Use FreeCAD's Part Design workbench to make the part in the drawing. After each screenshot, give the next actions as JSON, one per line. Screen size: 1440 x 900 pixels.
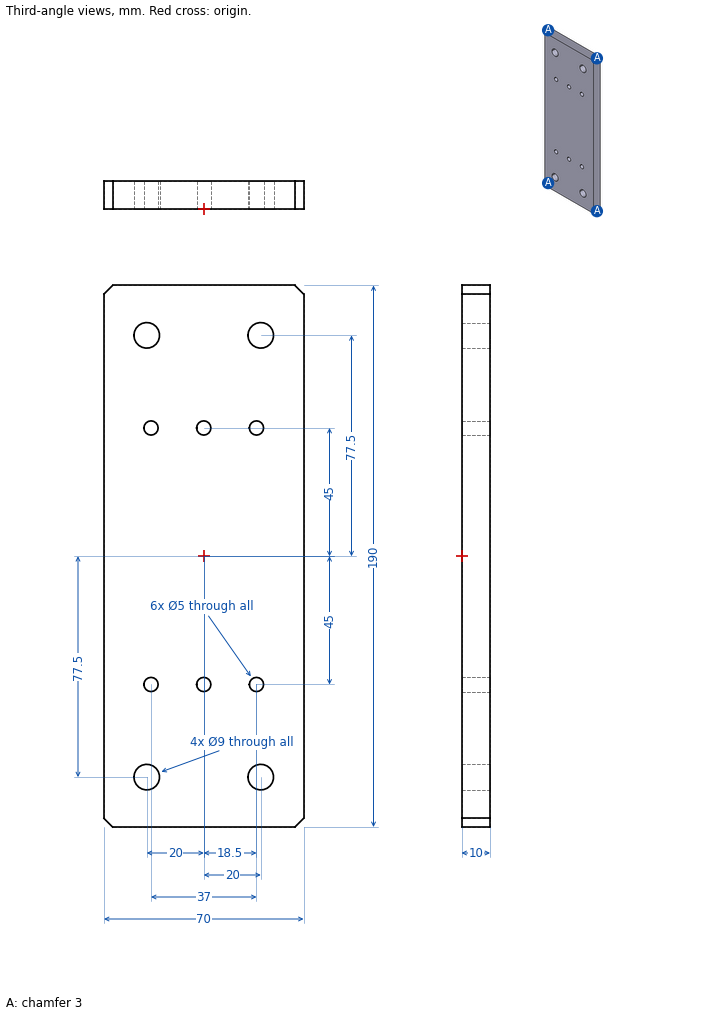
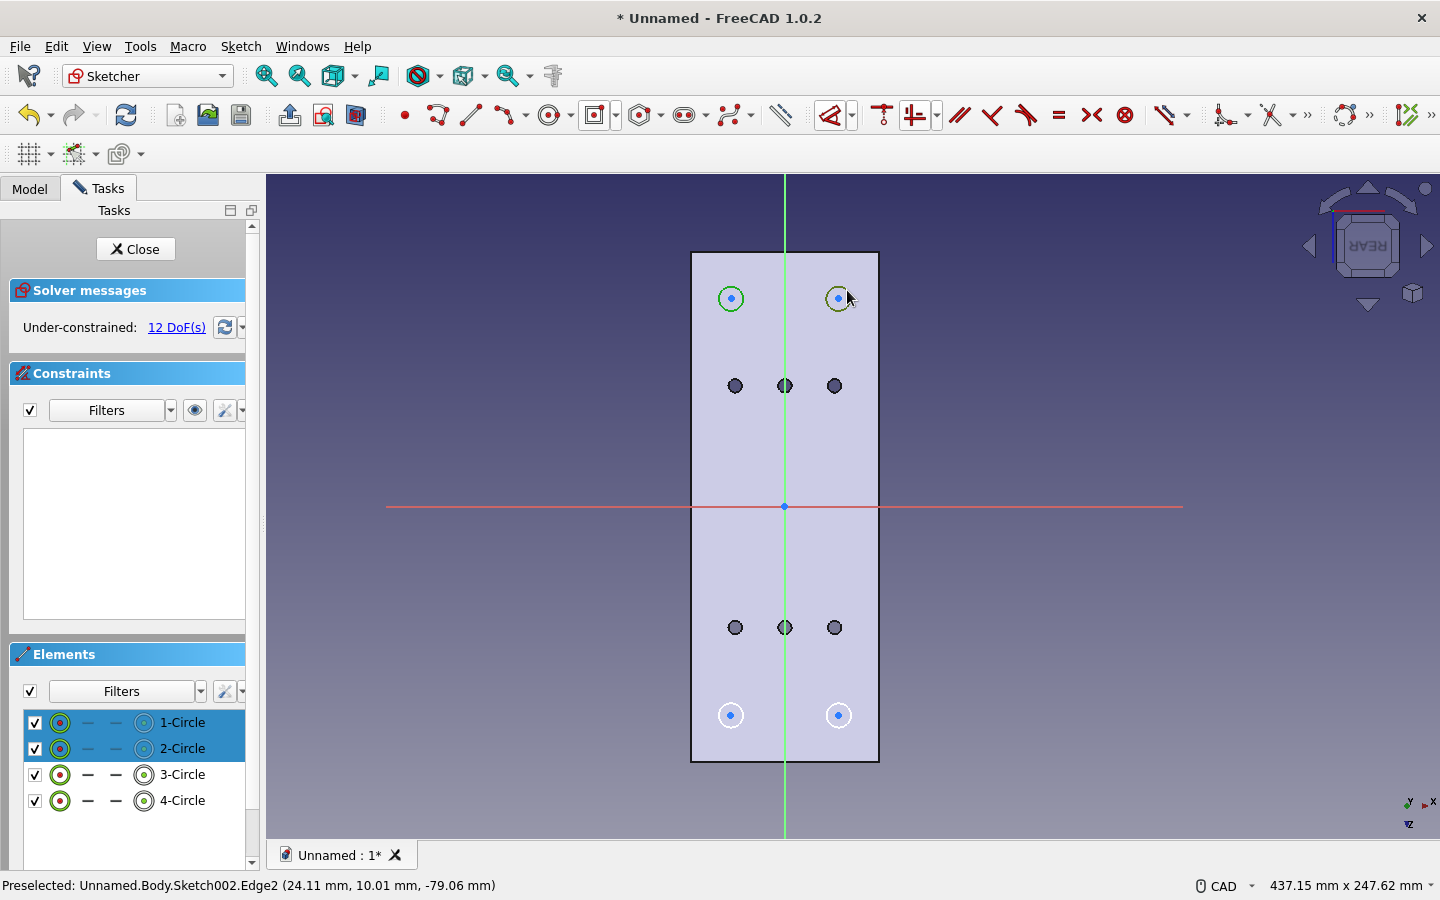
{"action": "left_click", "coordinate": [847, 707]}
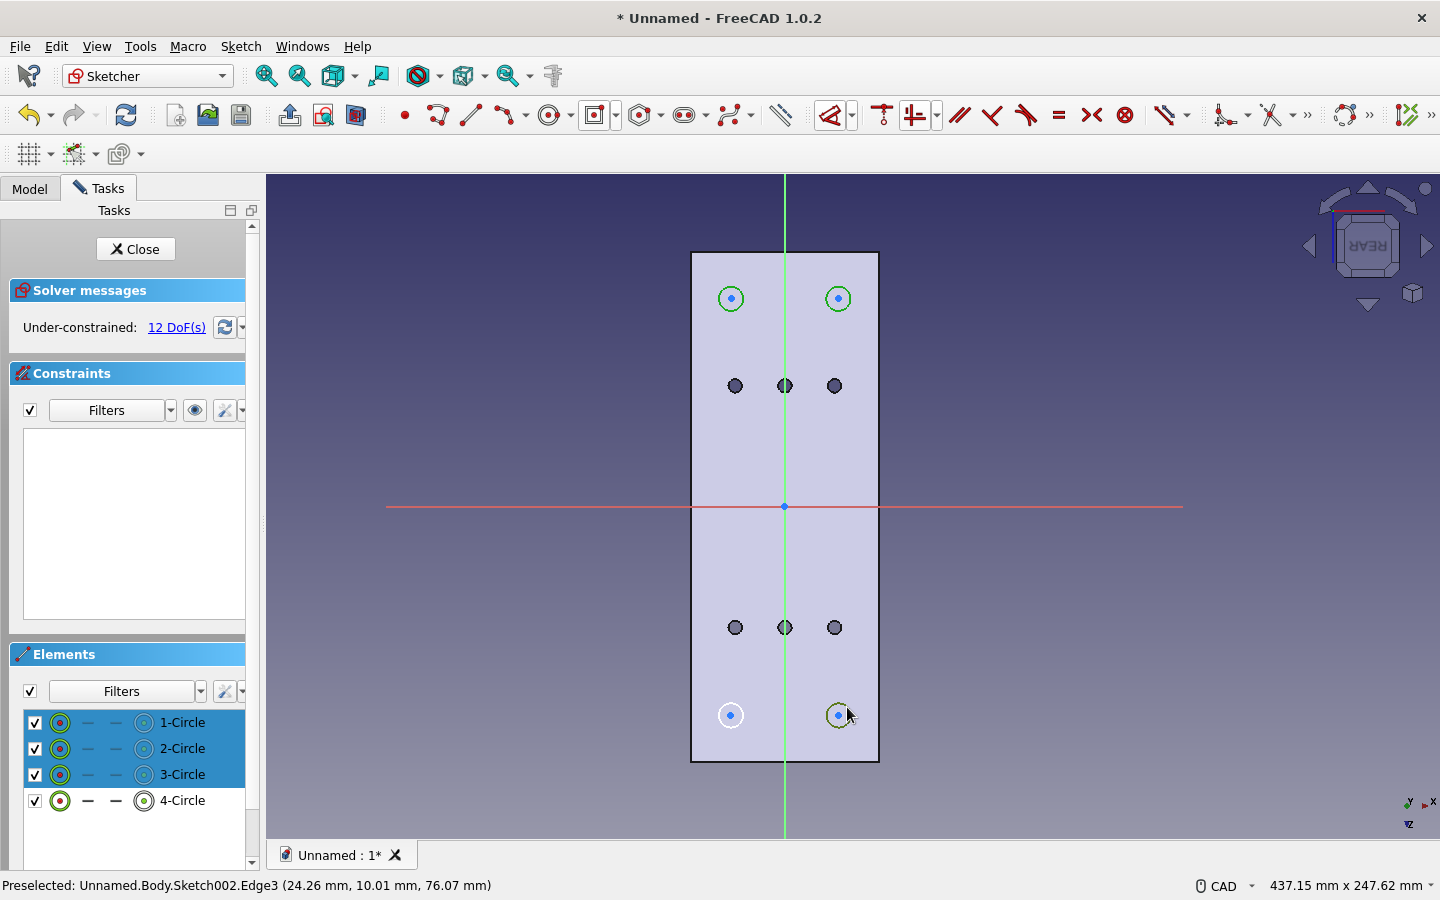
{"action": "left_click", "coordinate": [739, 707]}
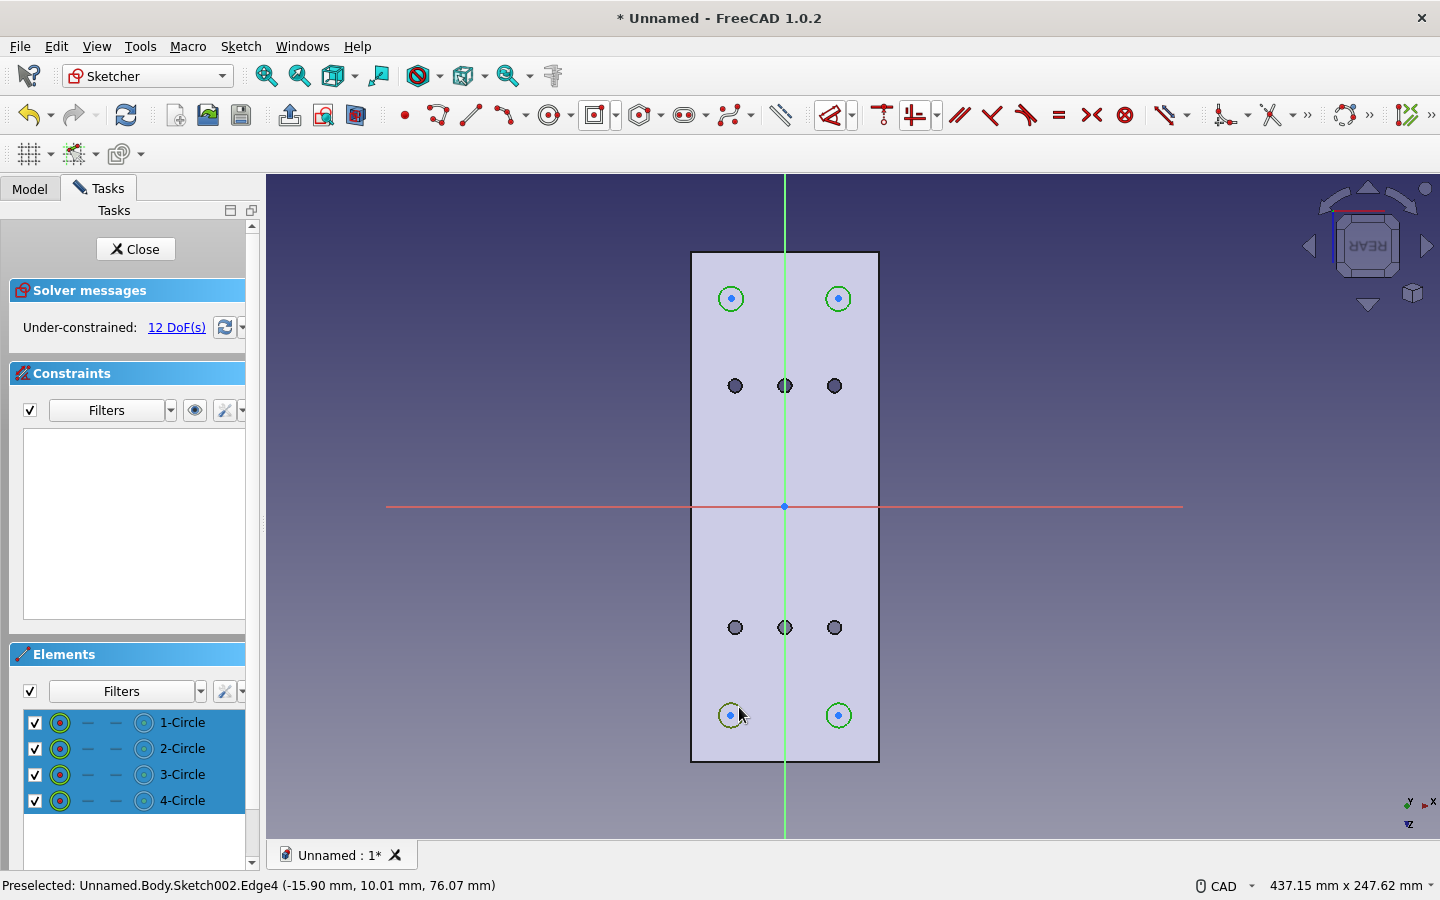
{"action": "left_click", "coordinate": [1059, 116]}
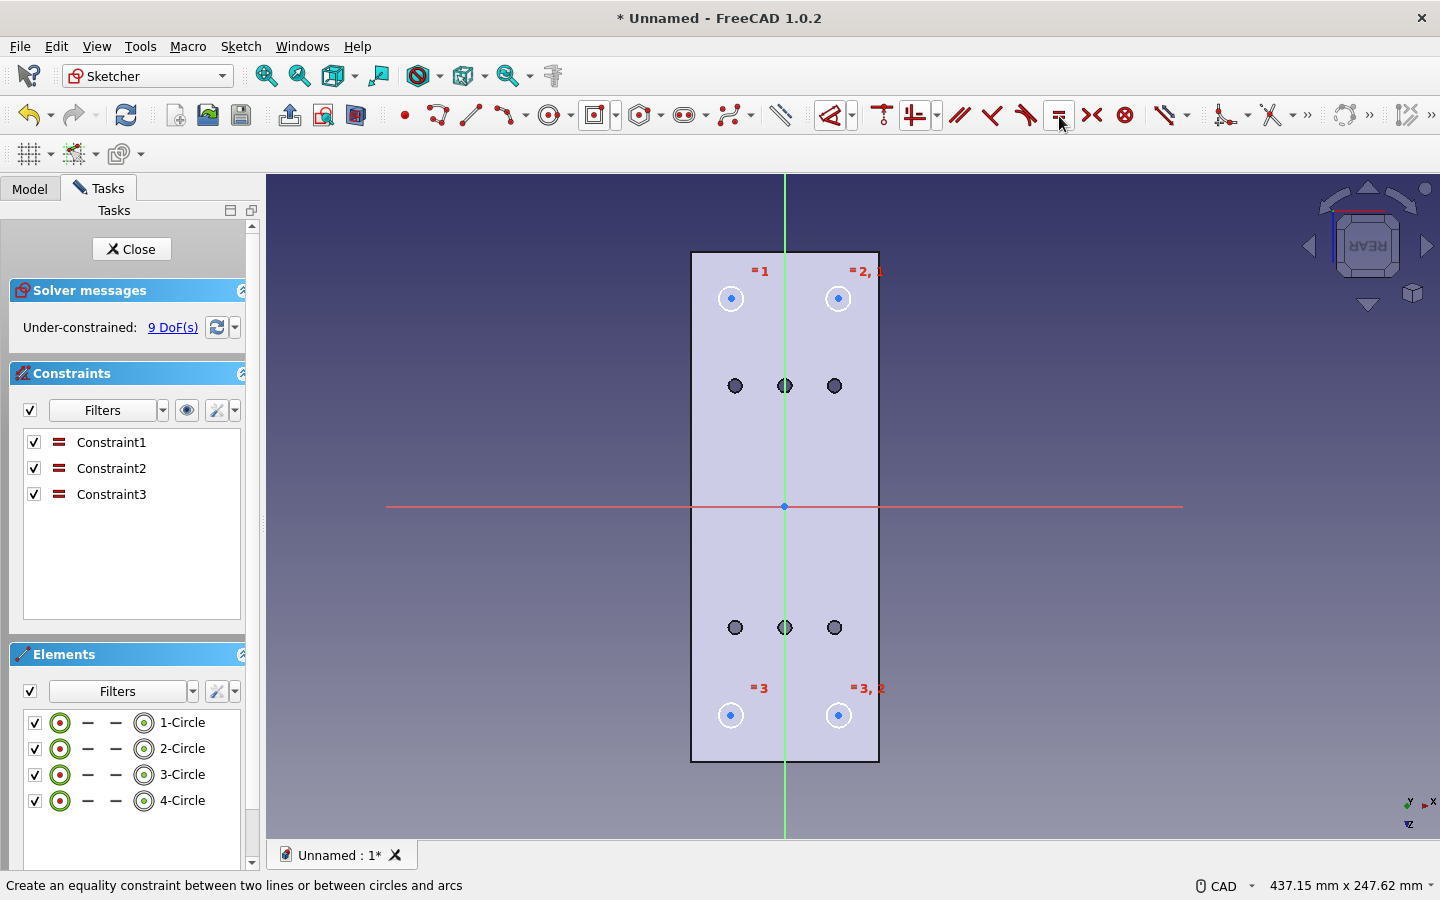
{"action": "left_click", "coordinate": [731, 299]}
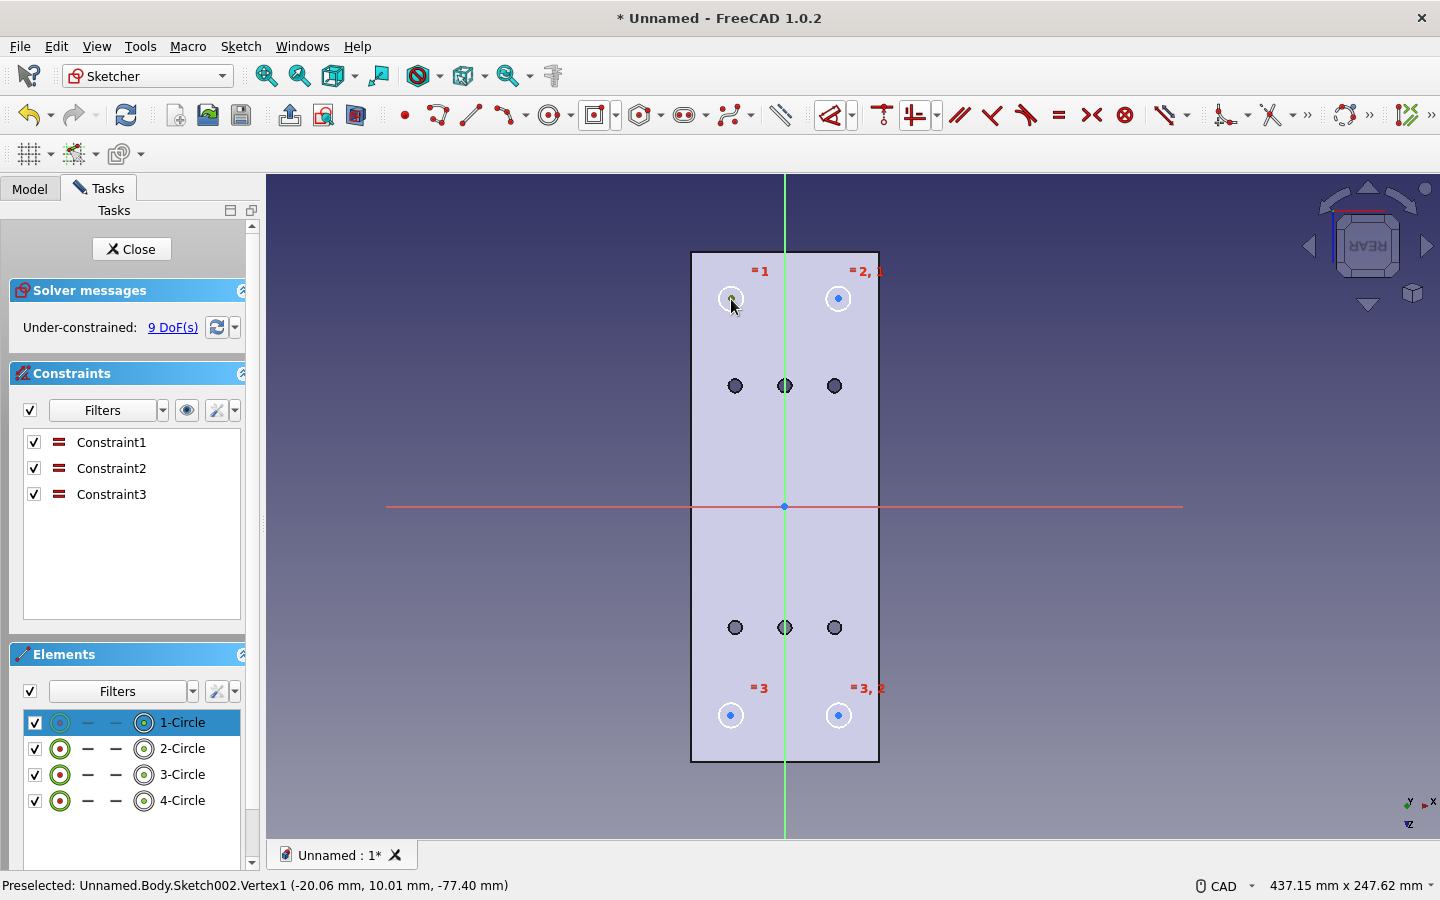
{"action": "left_click", "coordinate": [838, 299]}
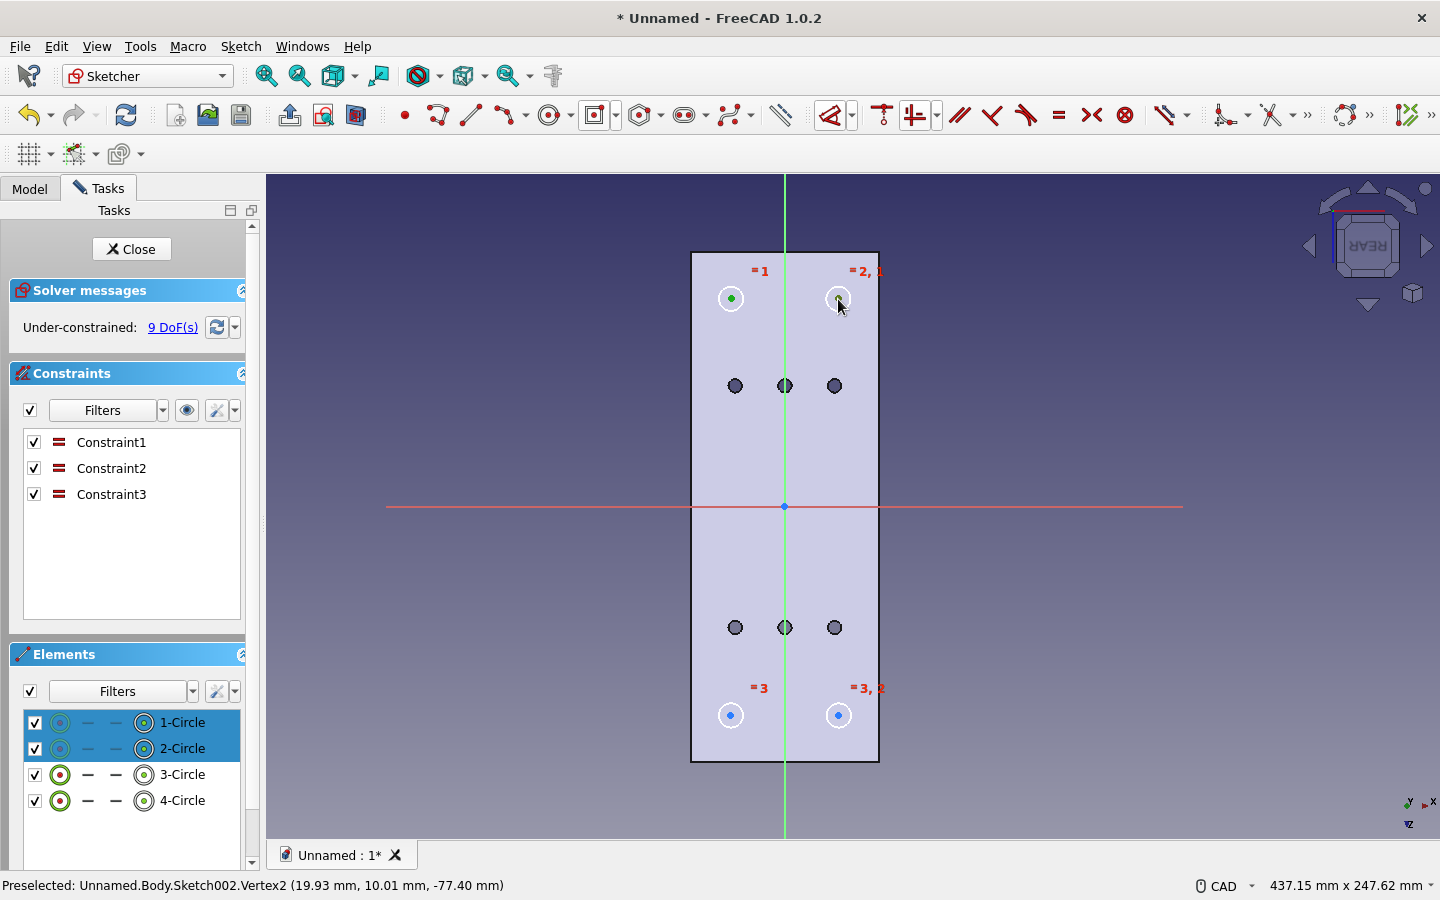
{"action": "key", "text": "h"}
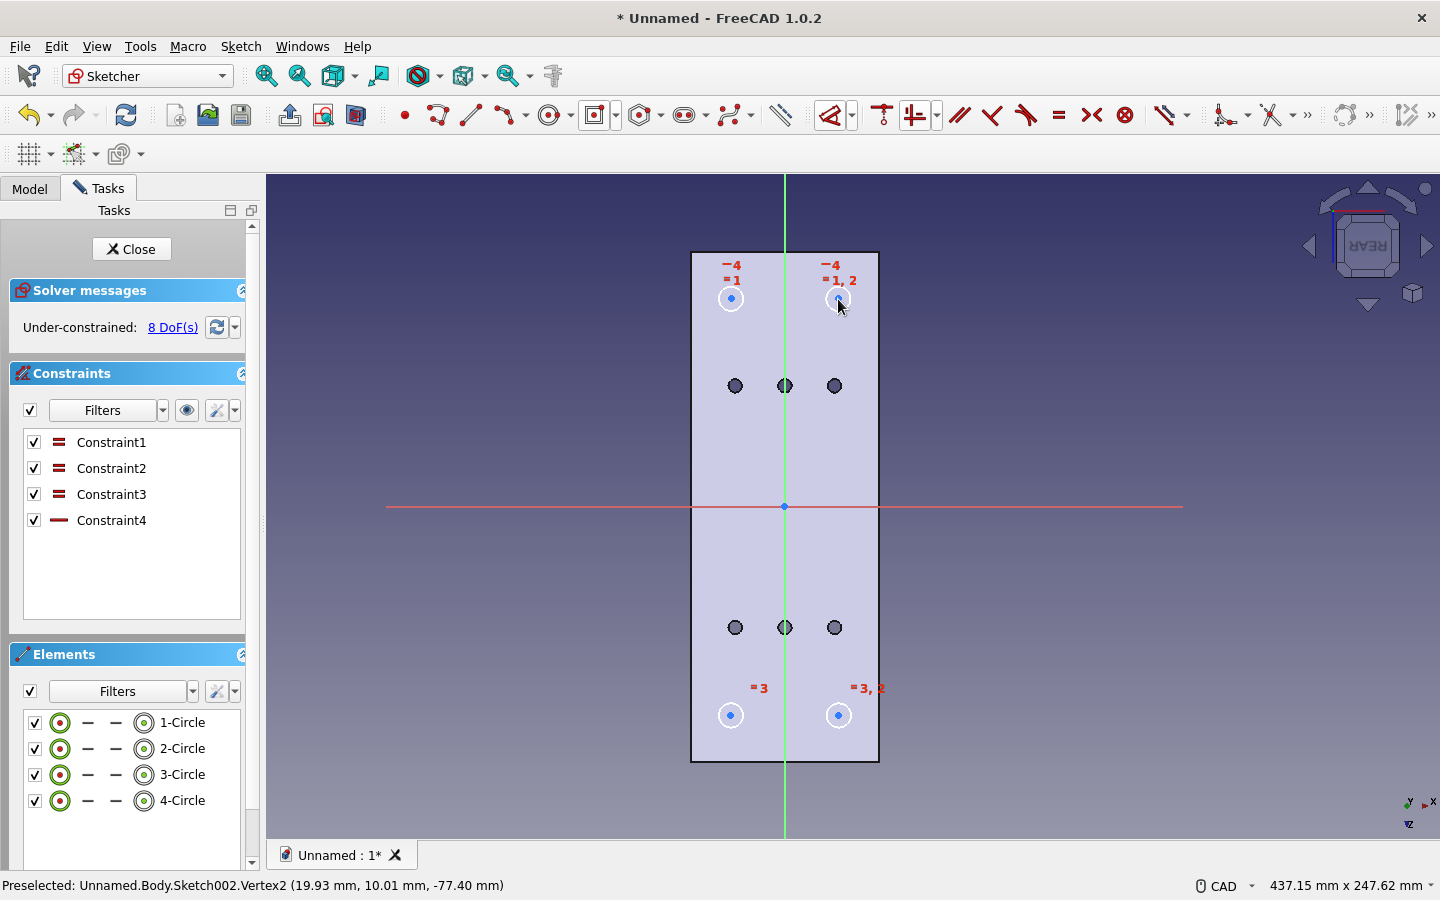
{"action": "left_click", "coordinate": [838, 299]}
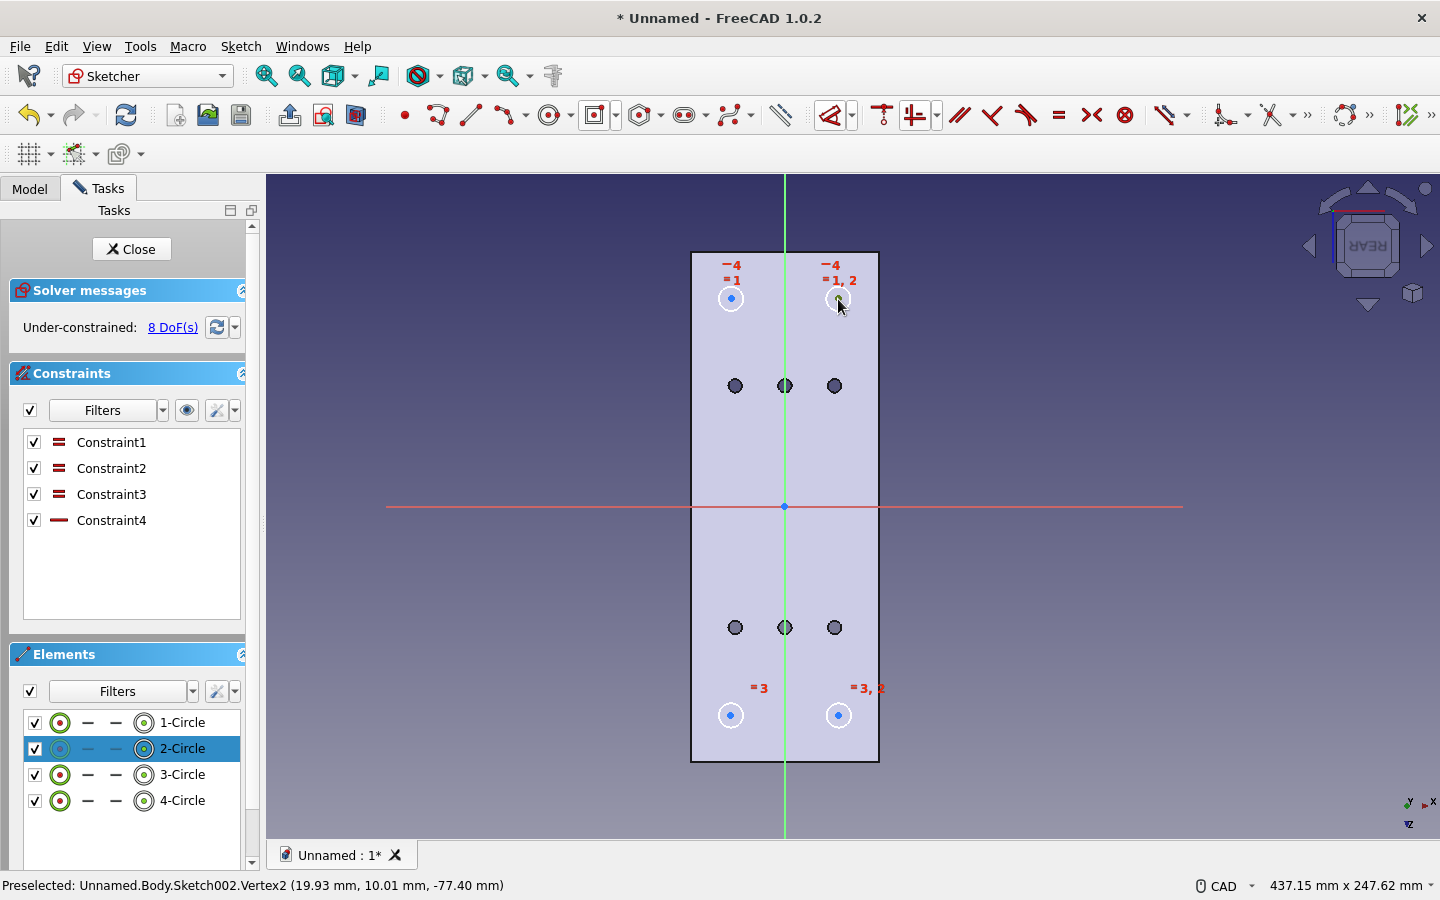
{"action": "left_click", "coordinate": [839, 715]}